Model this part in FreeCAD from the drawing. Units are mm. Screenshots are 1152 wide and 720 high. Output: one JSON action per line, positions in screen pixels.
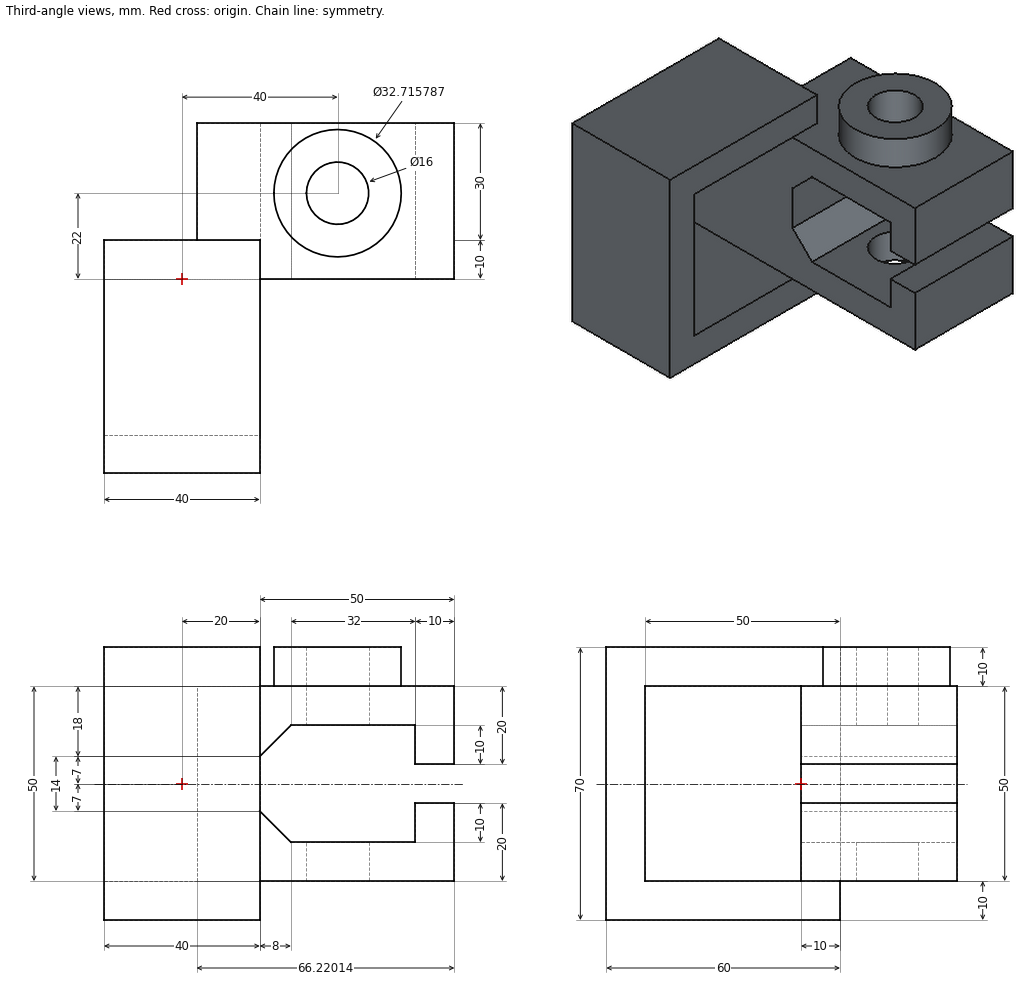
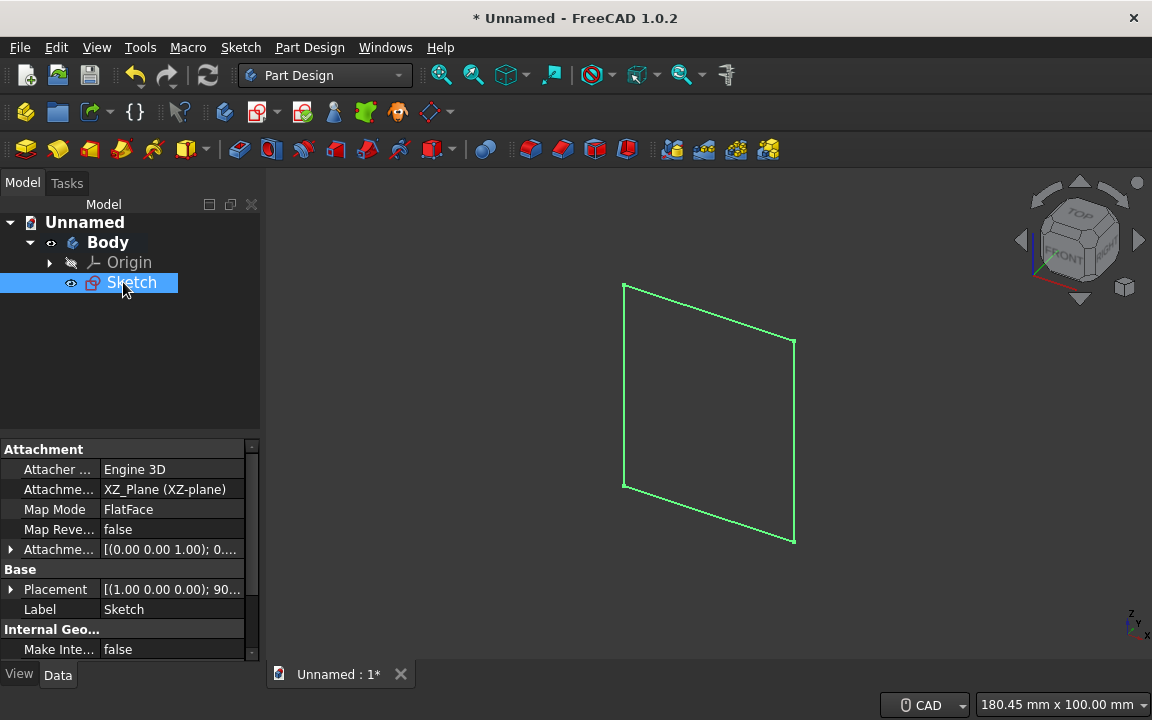
{"action": "left_click", "coordinate": [26, 150]}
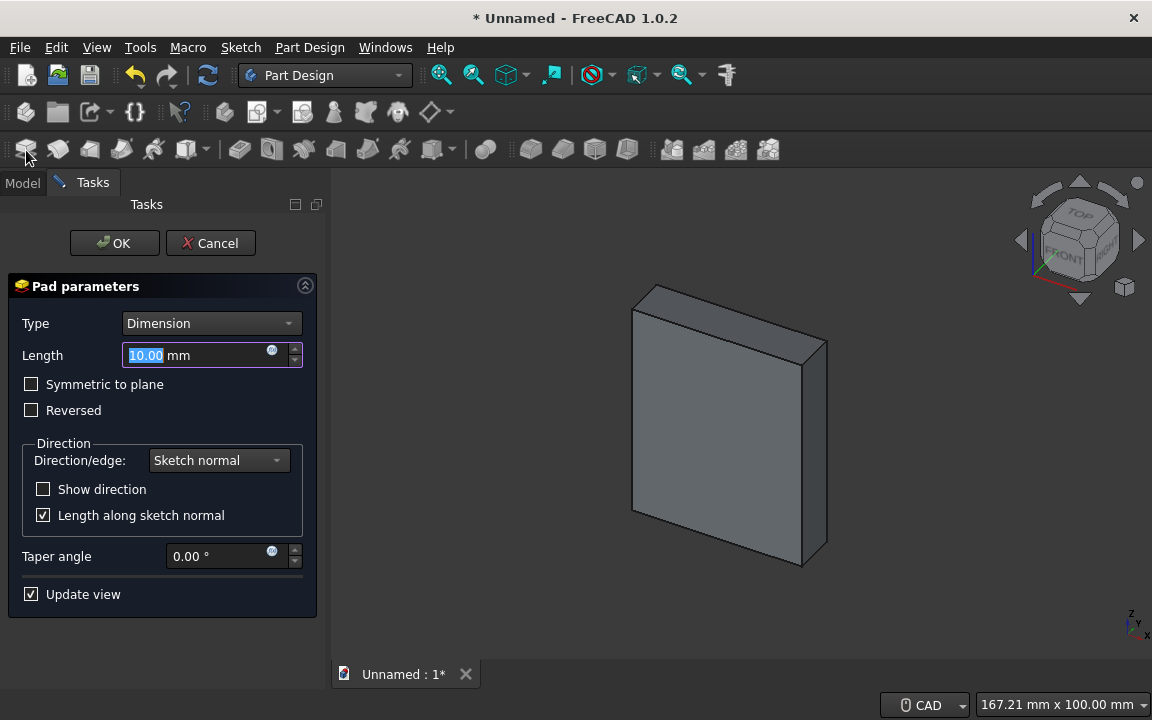
{"action": "type", "text": "10"}
{"action": "key", "text": "Tab"}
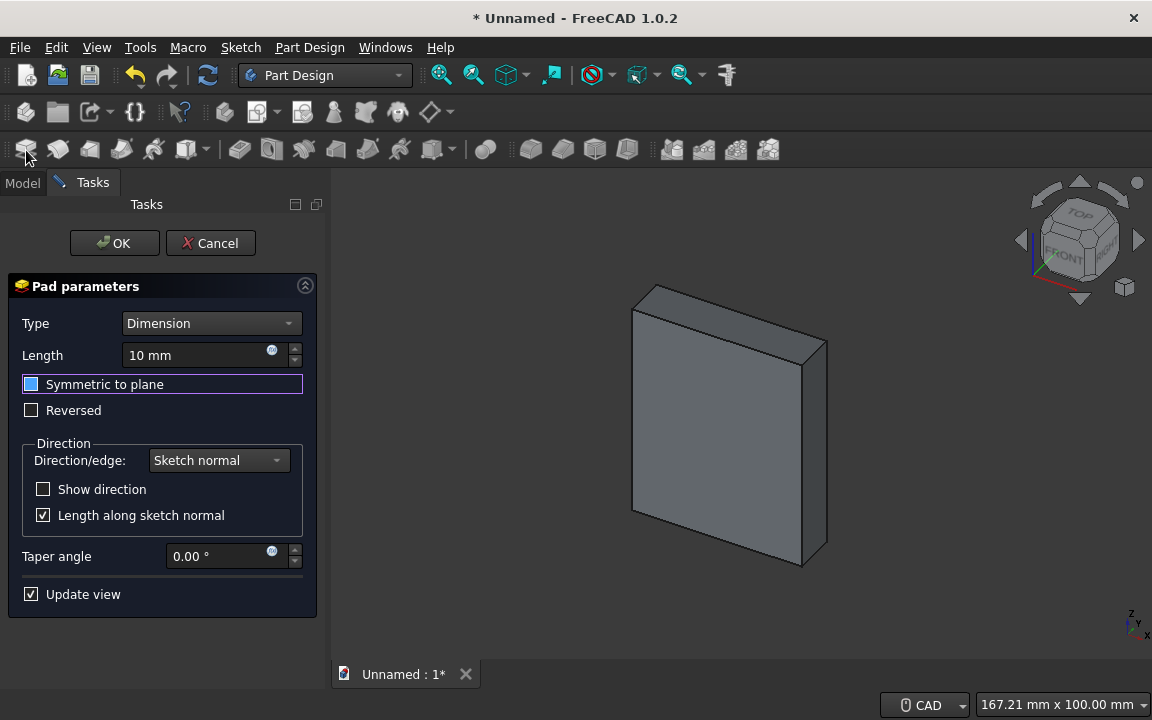
{"action": "left_click", "coordinate": [30, 410]}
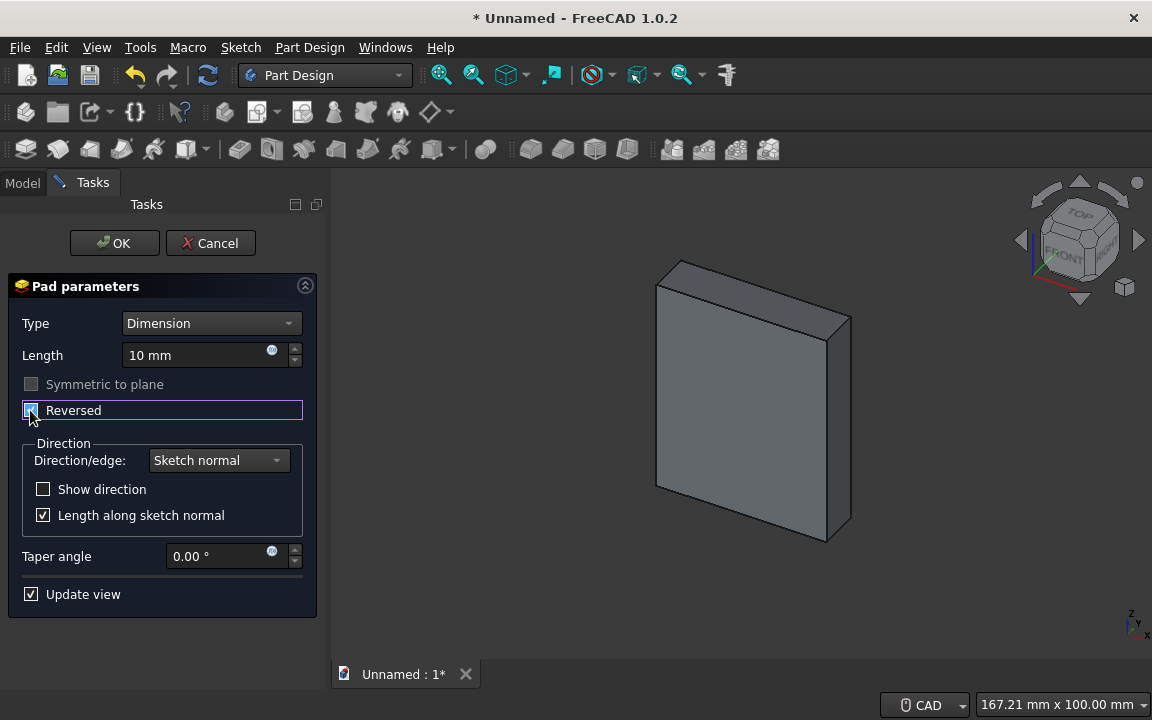
{"action": "left_click", "coordinate": [115, 243]}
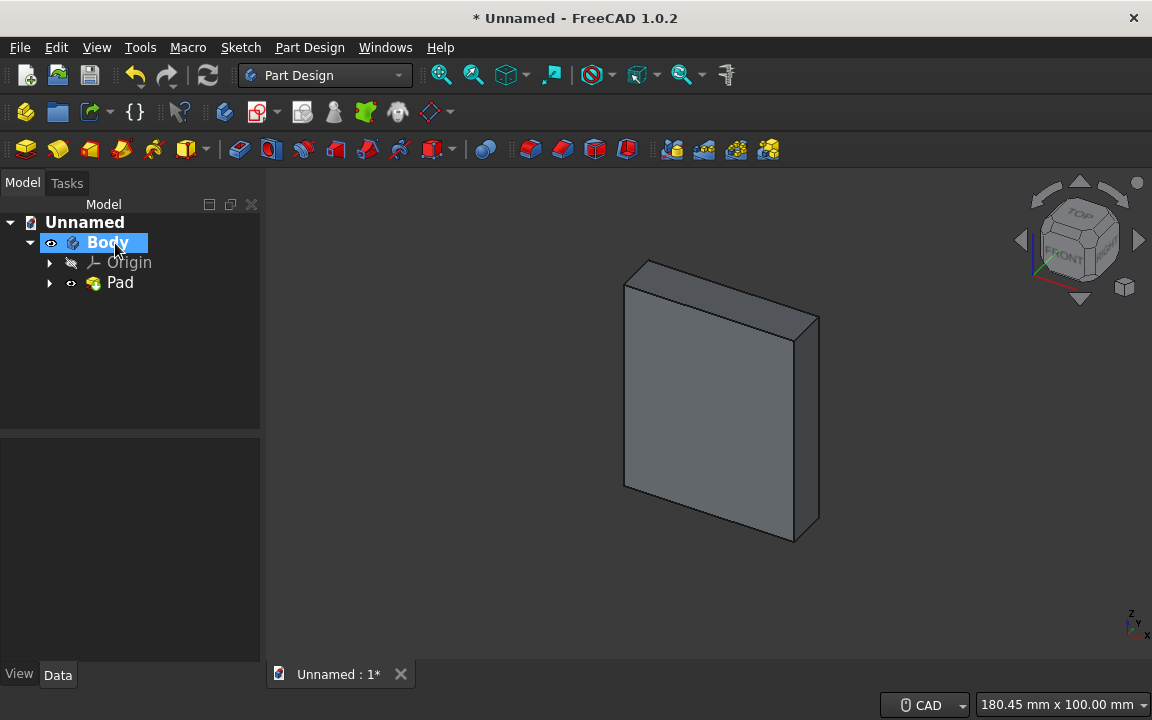
{"action": "key", "text": "4"}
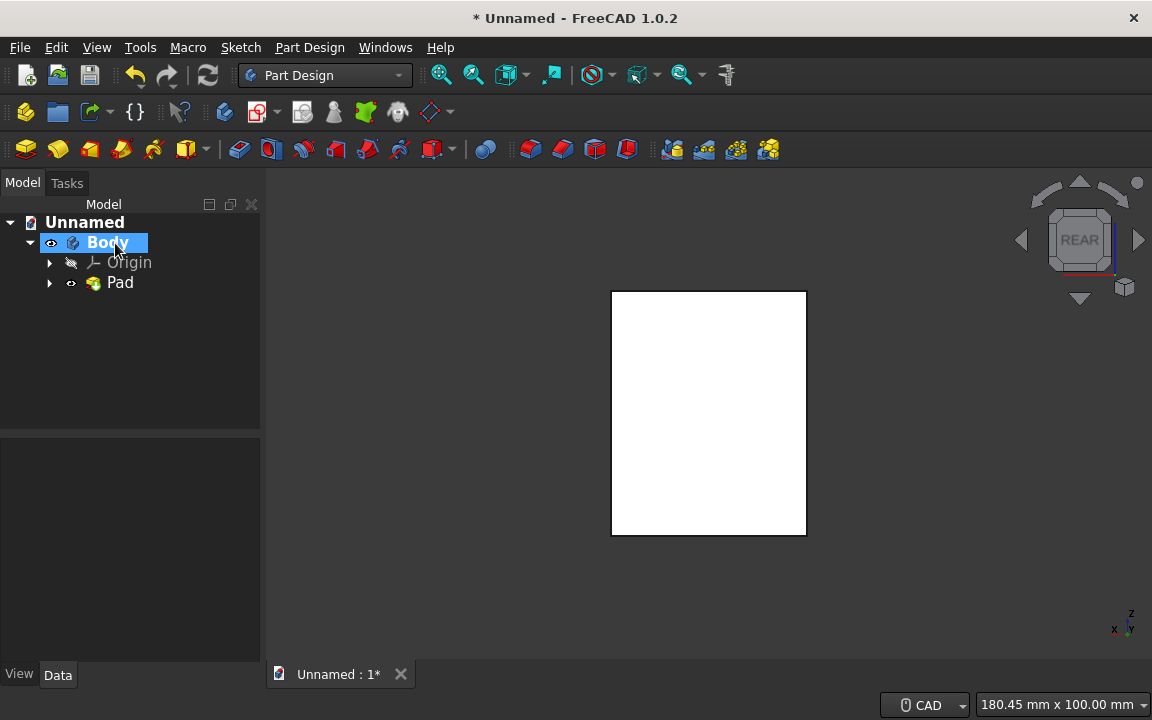
{"action": "left_click", "coordinate": [709, 412]}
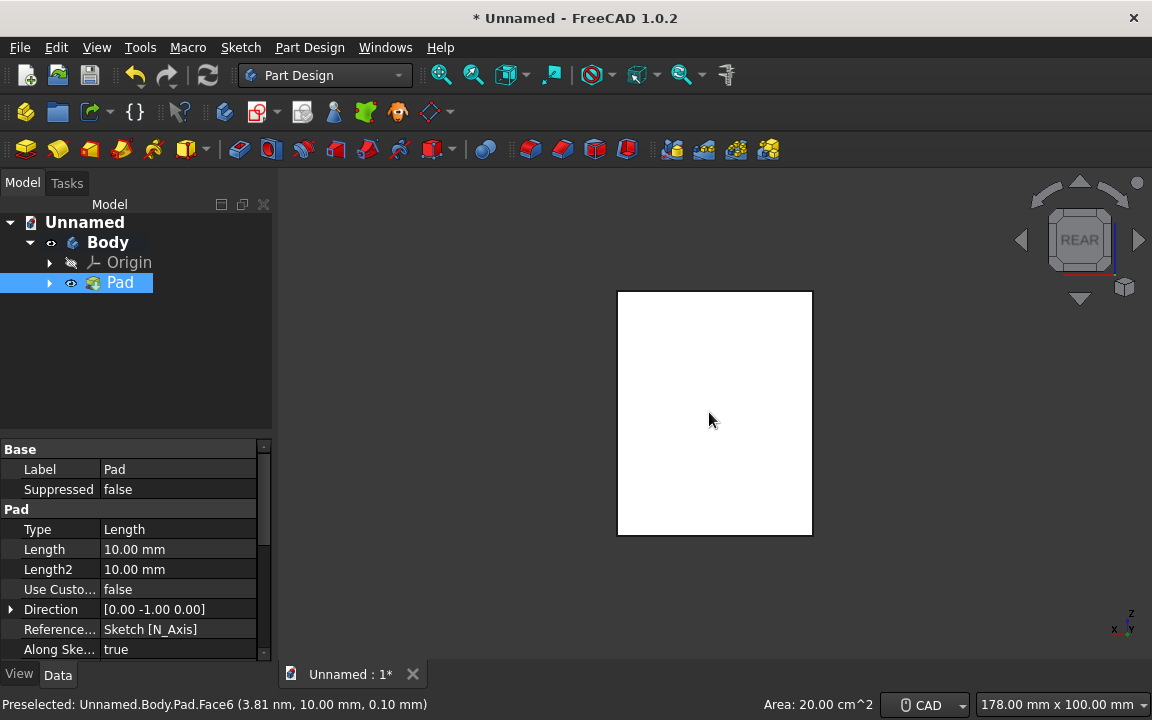
{"action": "left_click", "coordinate": [258, 112]}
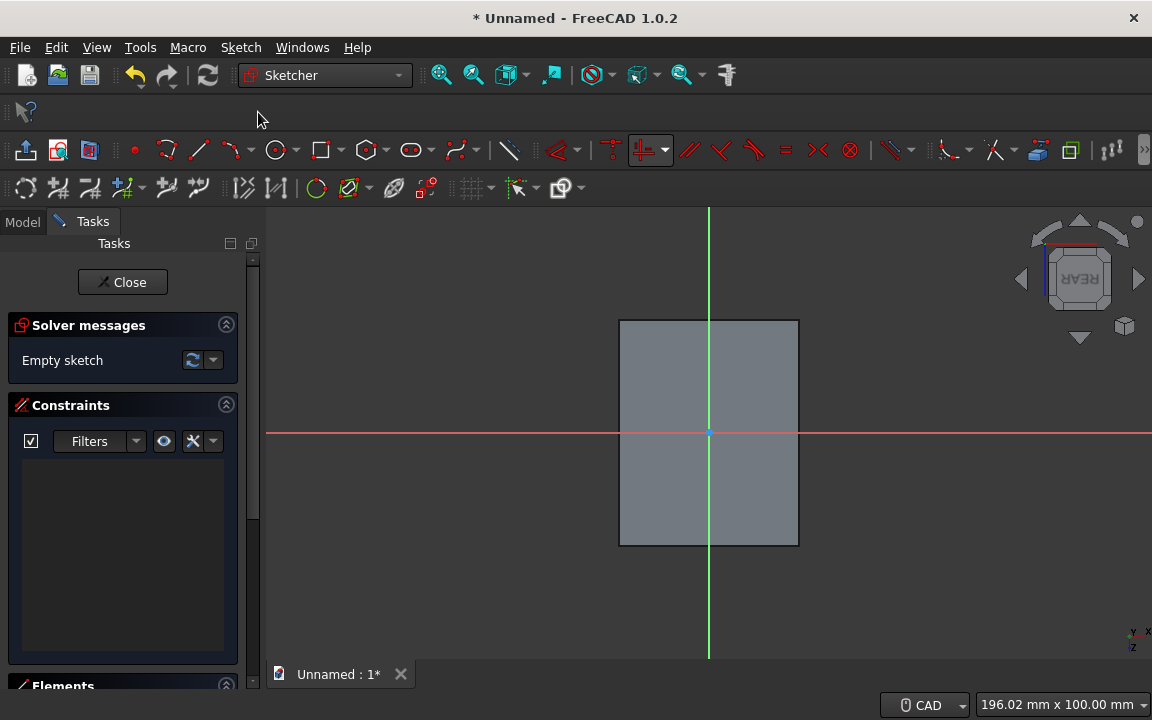
{"action": "scroll", "coordinate": [294, 433], "scroll_direction": "down", "scroll_amount": 1}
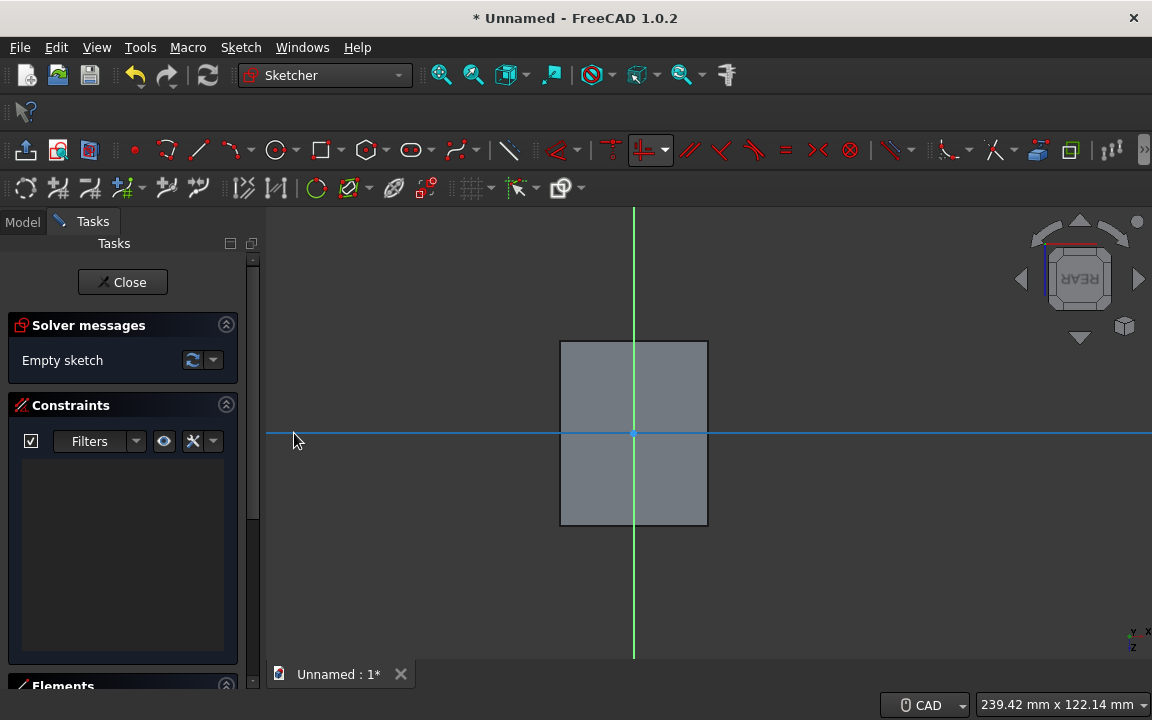
{"action": "scroll", "coordinate": [987, 433], "scroll_direction": "up", "scroll_amount": 2}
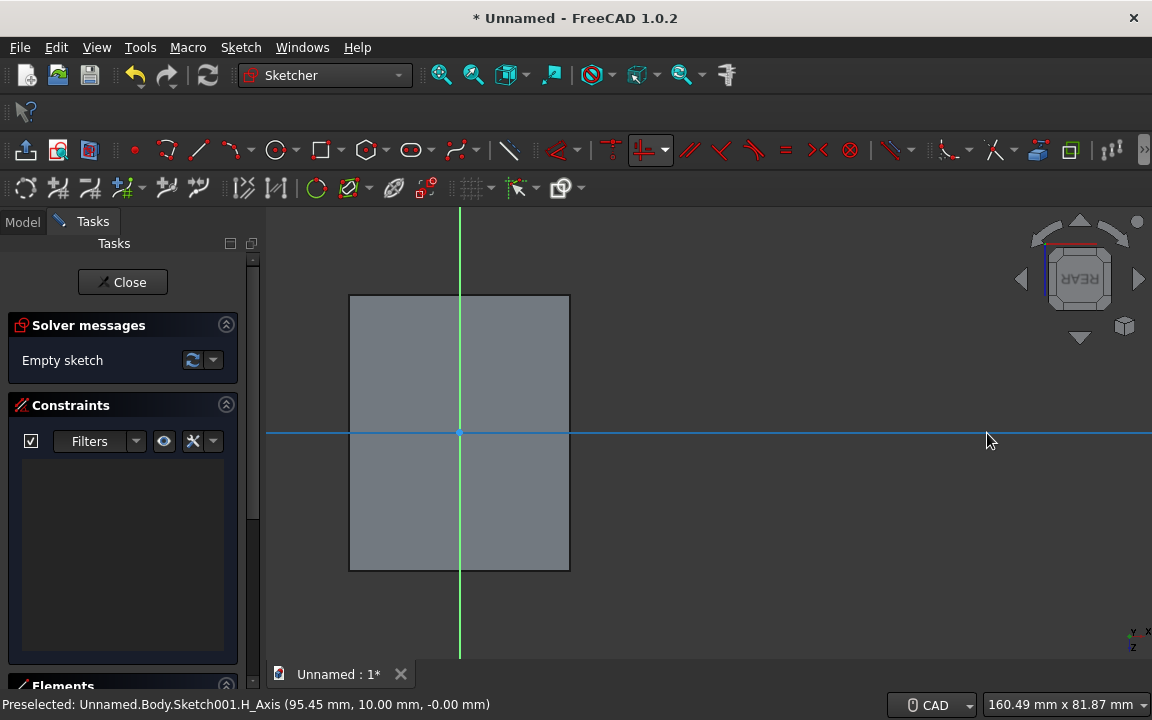
{"action": "left_click", "coordinate": [168, 150]}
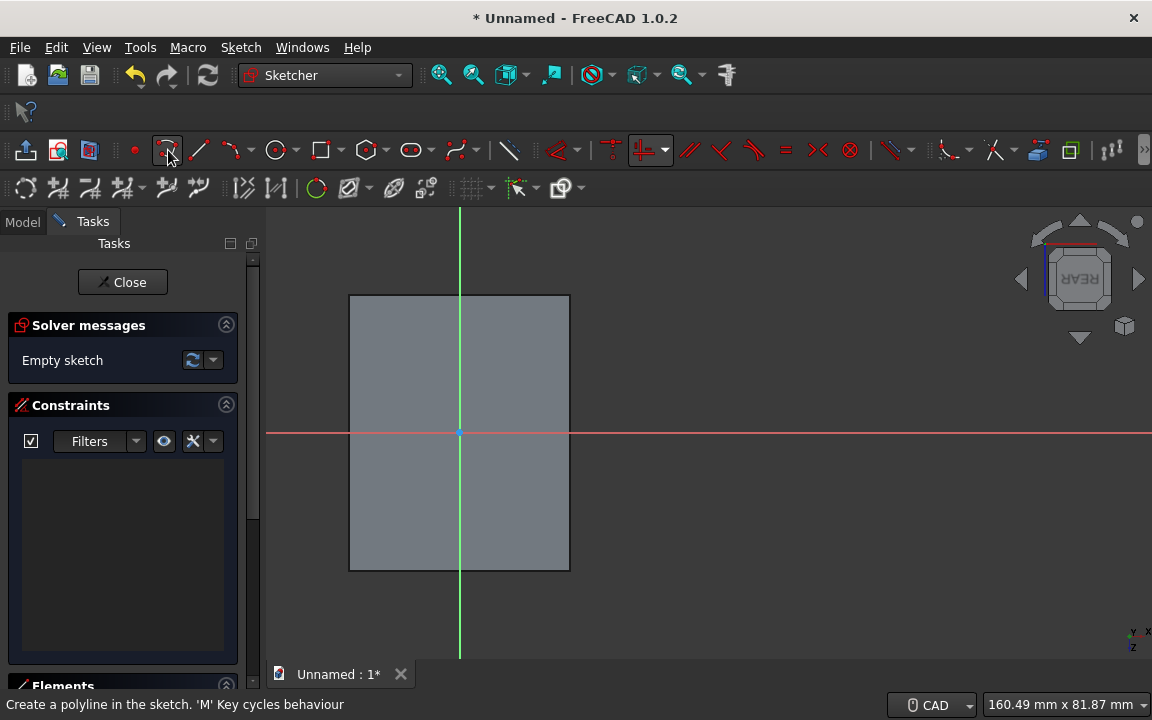
{"action": "left_click", "coordinate": [570, 472]}
{"action": "left_click", "coordinate": [570, 571]}
{"action": "left_click", "coordinate": [846, 571]}
{"action": "left_click", "coordinate": [846, 460]}
{"action": "left_click", "coordinate": [791, 460]}
{"action": "left_click", "coordinate": [791, 516]}
{"action": "left_click", "coordinate": [614, 516]}
{"action": "left_click", "coordinate": [570, 473]}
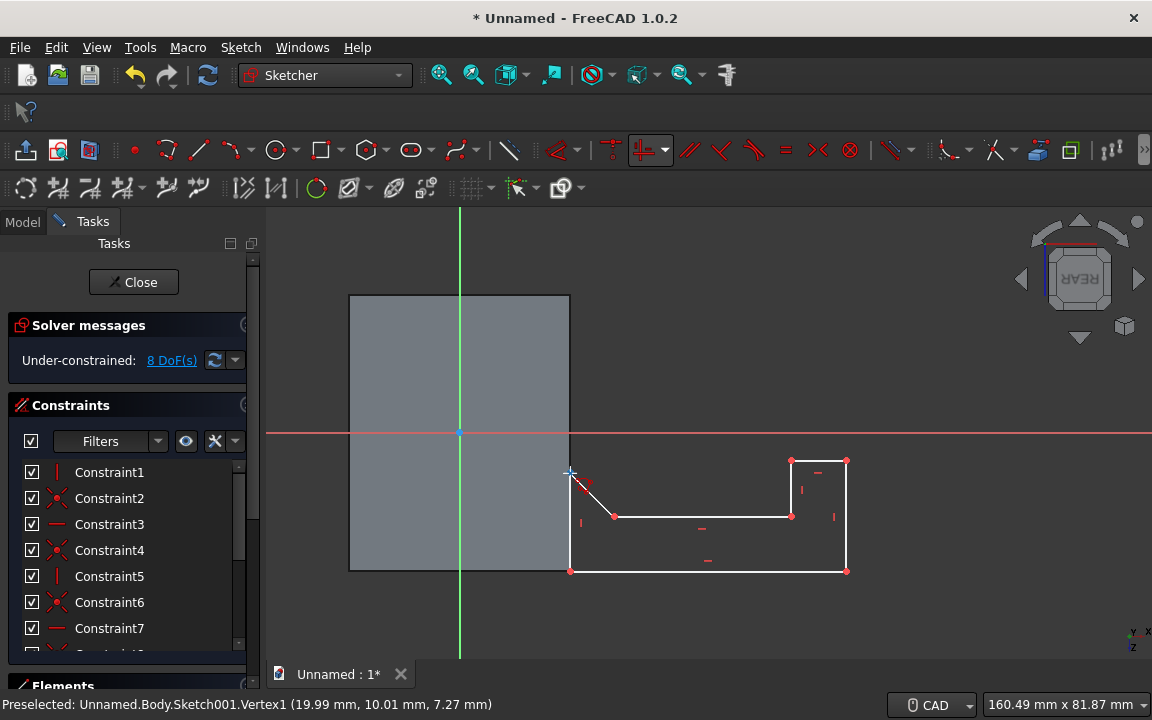
{"action": "left_click", "coordinate": [570, 394]}
{"action": "left_click", "coordinate": [614, 350]}
{"action": "left_click", "coordinate": [791, 350]}
{"action": "left_click", "coordinate": [791, 405]}
{"action": "left_click", "coordinate": [846, 405]}
{"action": "left_click", "coordinate": [846, 295]}
{"action": "left_click", "coordinate": [570, 295]}
{"action": "left_click", "coordinate": [570, 395]}
{"action": "key", "text": "Escape"}
{"action": "key", "text": "Escape"}